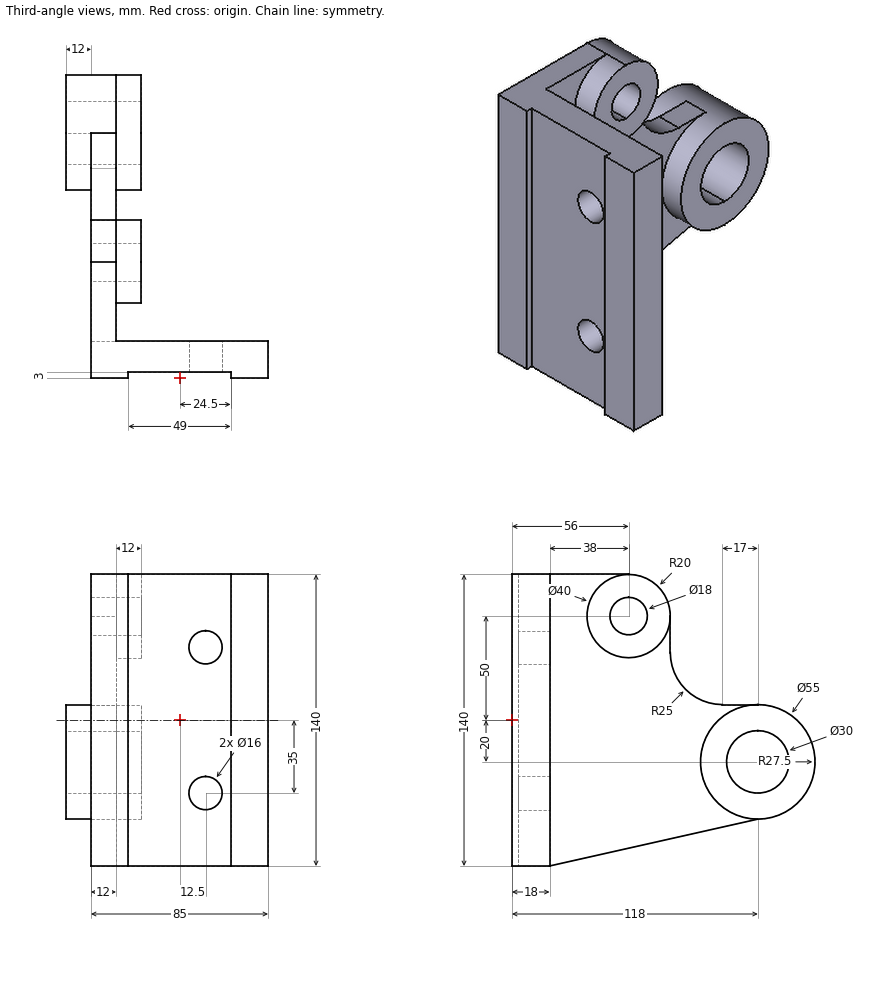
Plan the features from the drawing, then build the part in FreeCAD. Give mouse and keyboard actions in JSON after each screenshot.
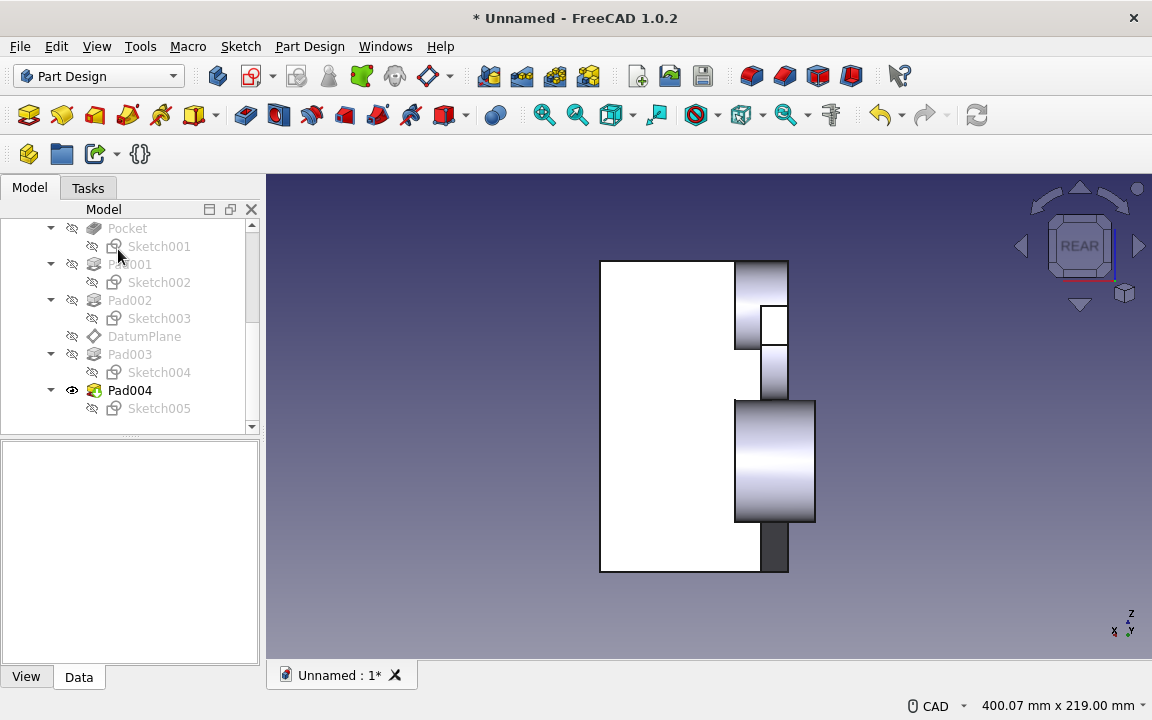
{"action": "left_click", "coordinate": [681, 371]}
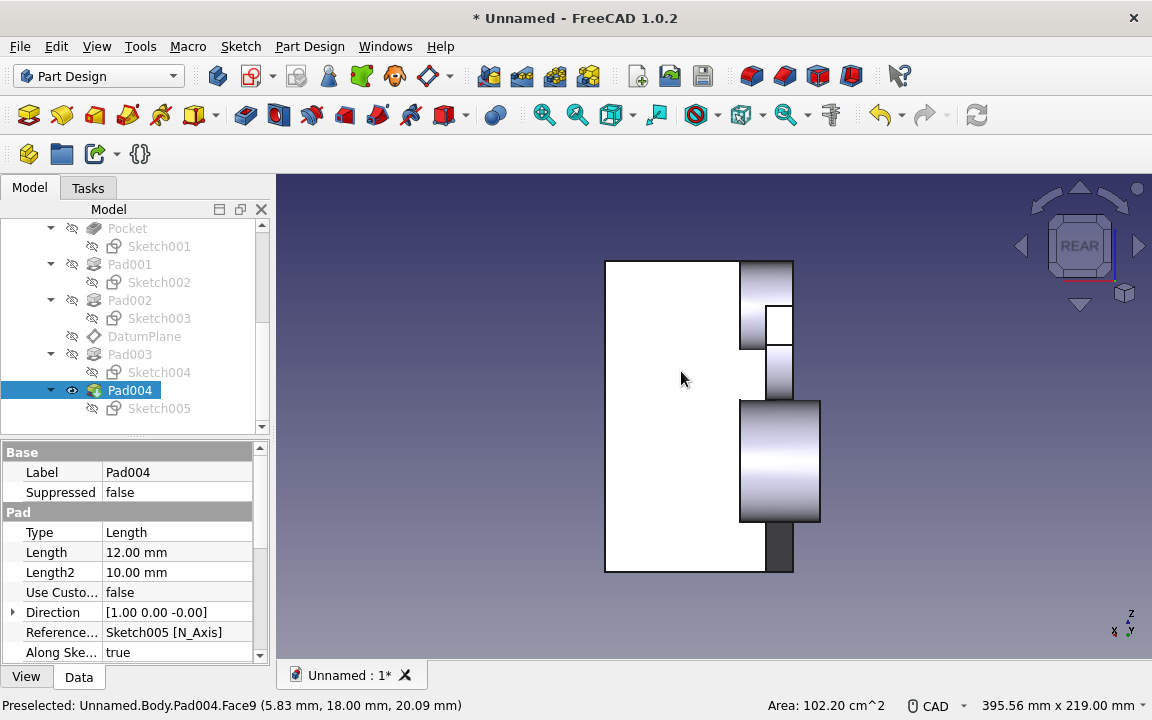
{"action": "left_click", "coordinate": [250, 76]}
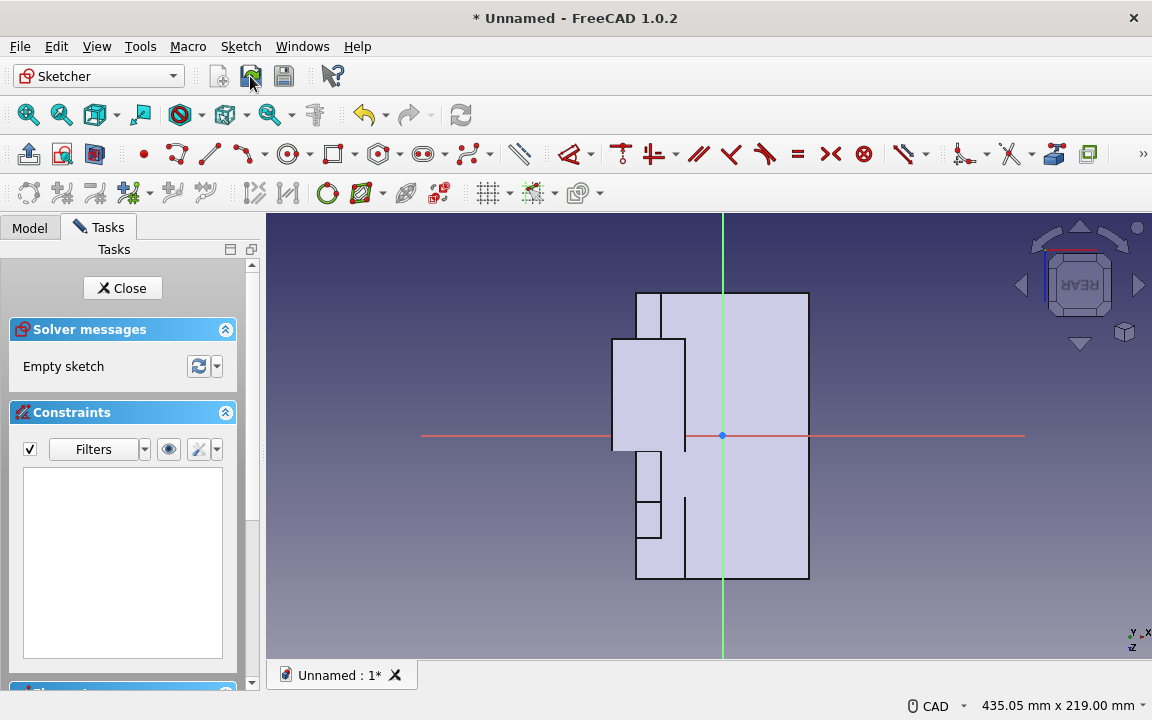
{"action": "left_click", "coordinate": [95, 154]}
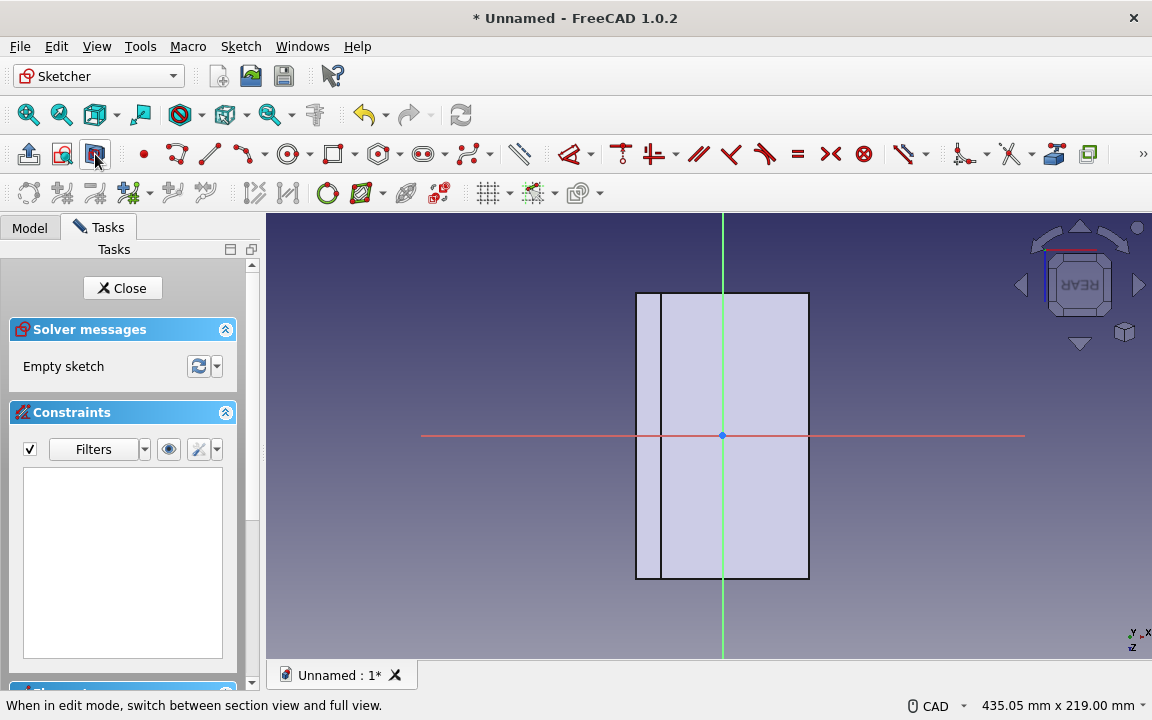
{"action": "scroll", "coordinate": [954, 436], "scroll_direction": "up", "scroll_amount": 2}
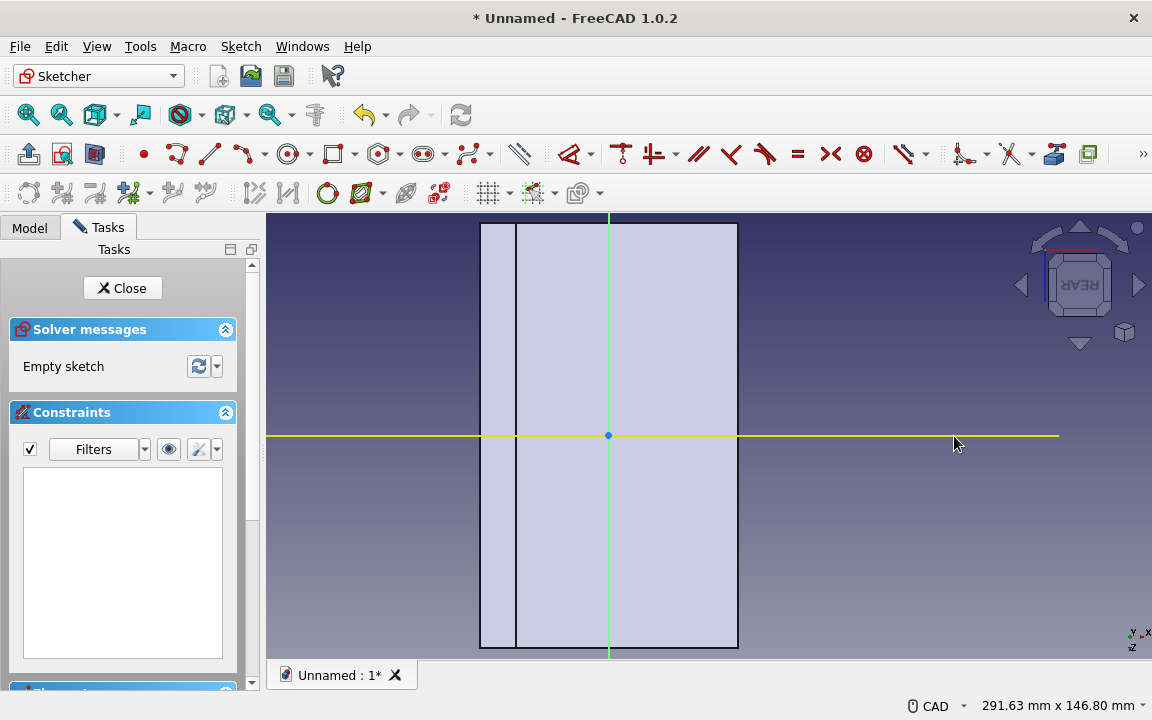
{"action": "key", "text": "g c"}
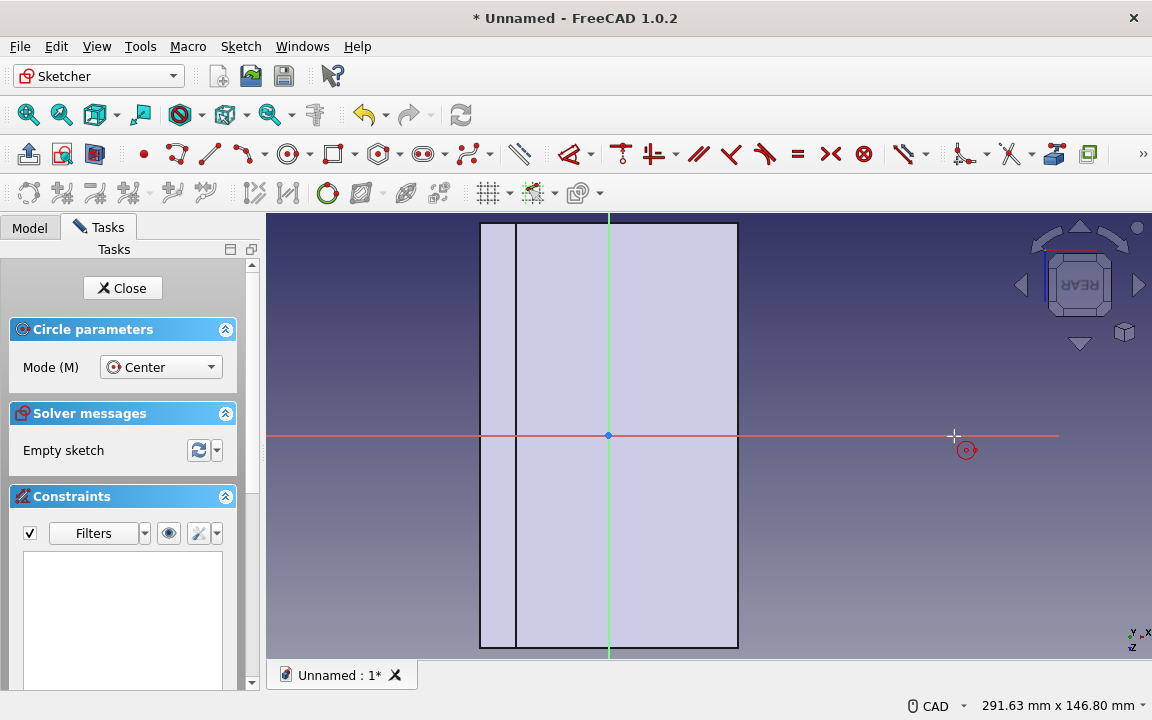
{"action": "left_click", "coordinate": [647, 329]}
{"action": "mouse_move", "coordinate": [664, 312]}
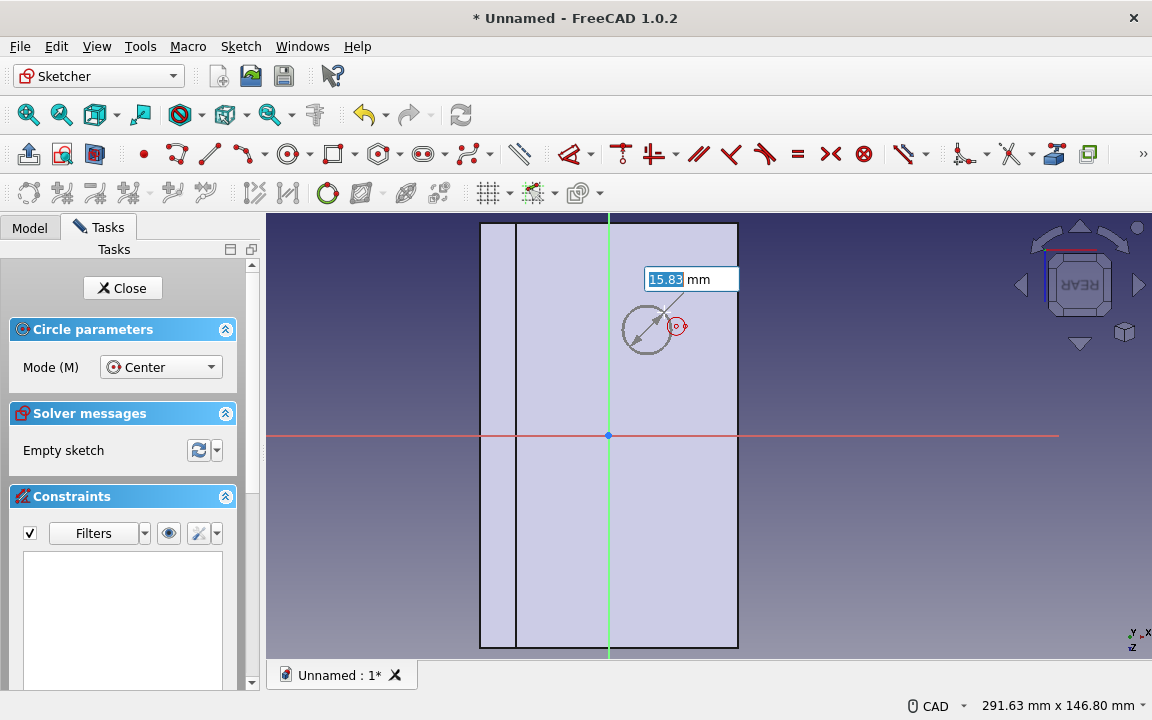
{"action": "type", "text": "16"}
{"action": "key", "text": "Return"}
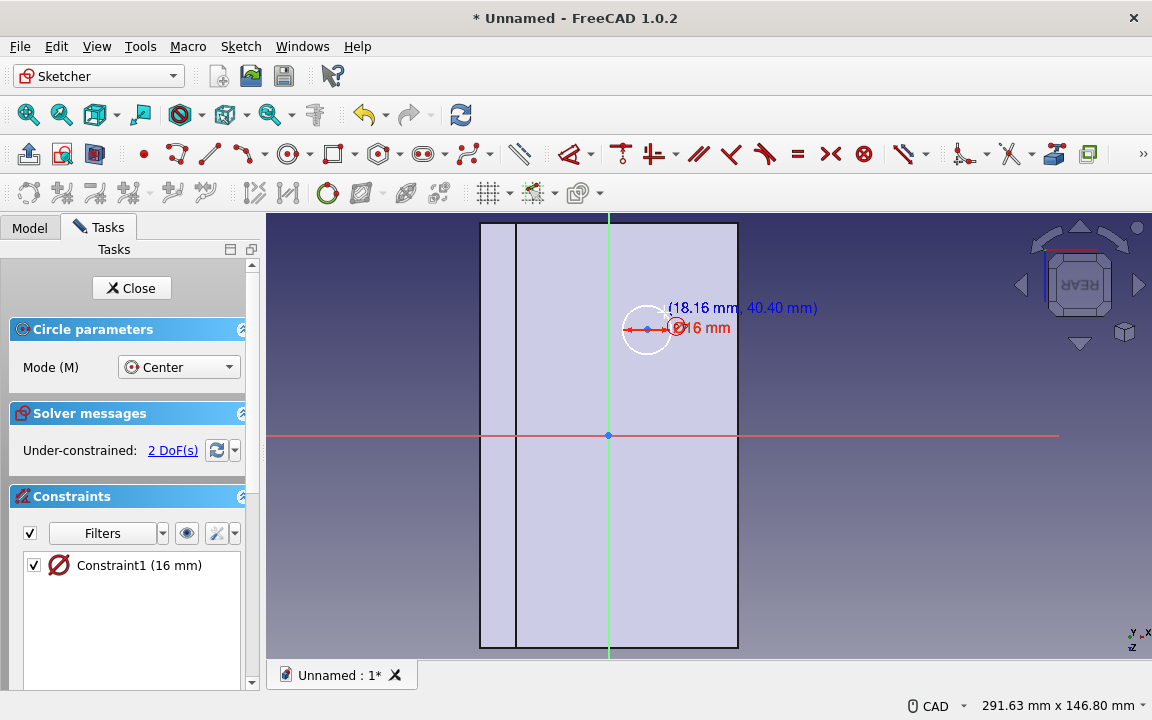
{"action": "left_click", "coordinate": [647, 542]}
{"action": "mouse_move", "coordinate": [664, 525]}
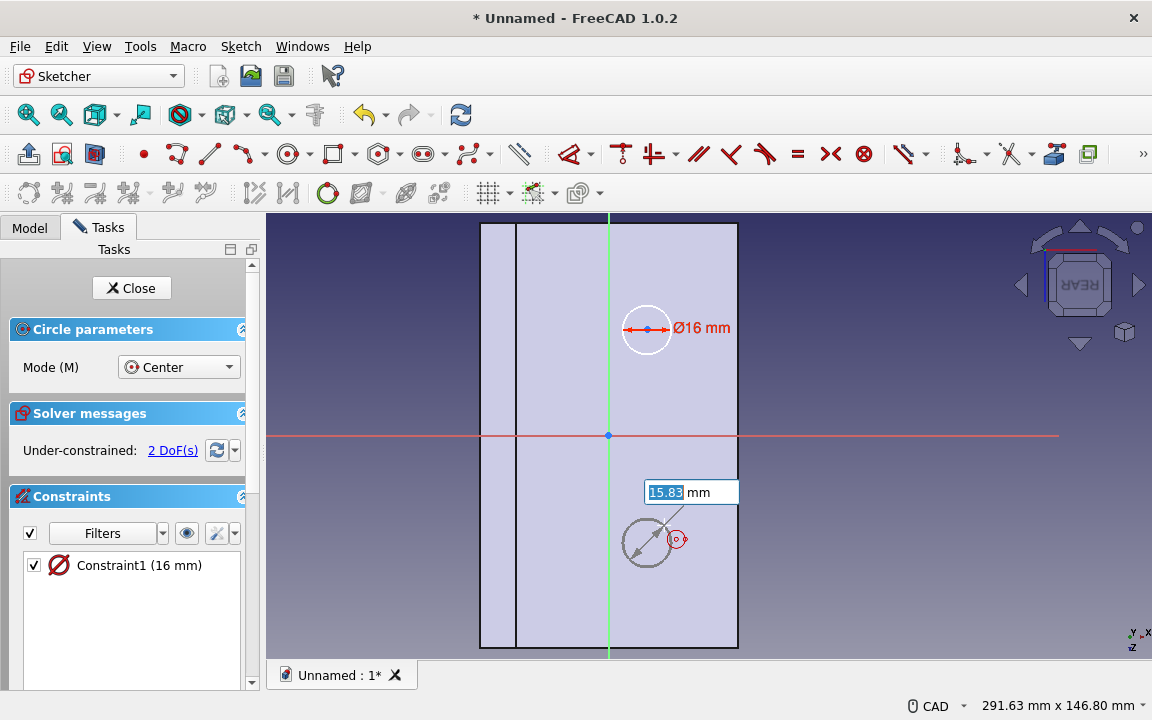
{"action": "type", "text": "16"}
{"action": "key", "text": "Return"}
{"action": "key", "text": "Escape"}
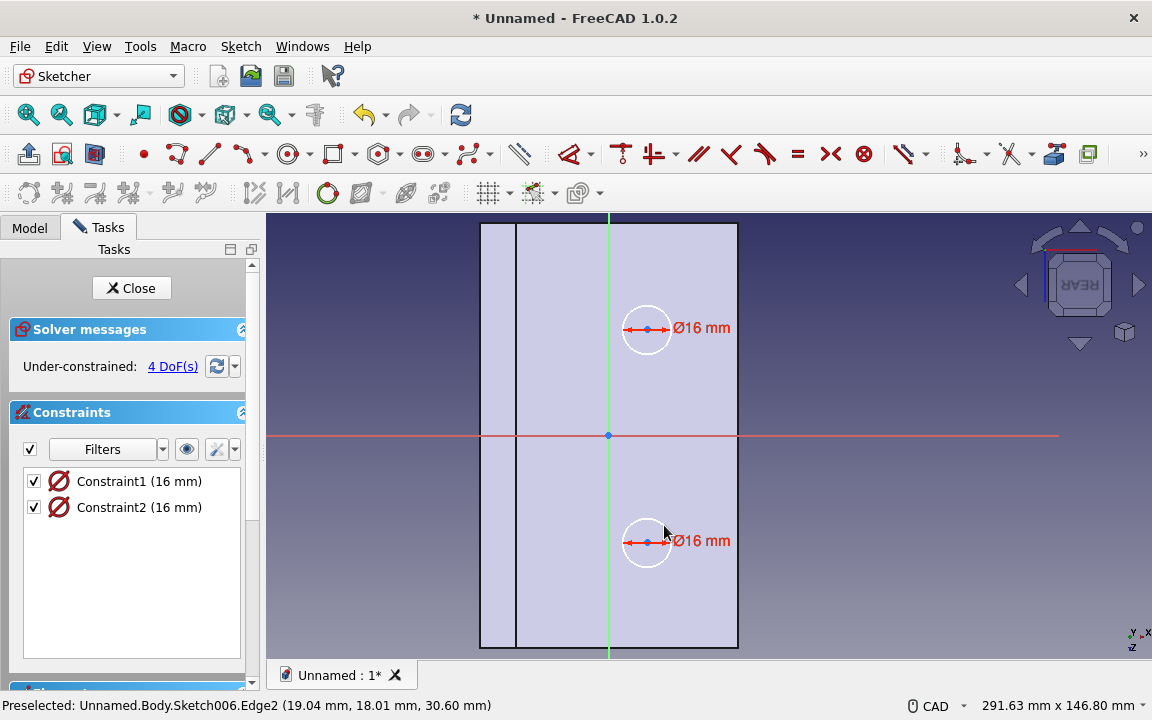
{"action": "left_click", "coordinate": [647, 330]}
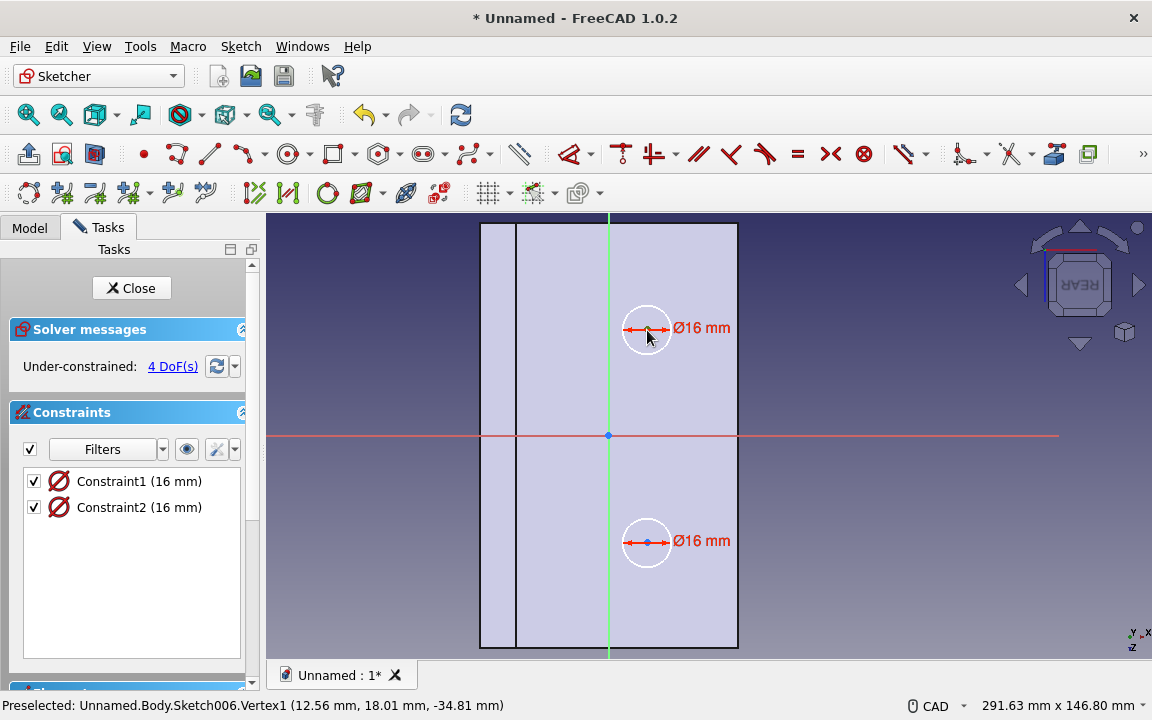
{"action": "left_click", "coordinate": [647, 543]}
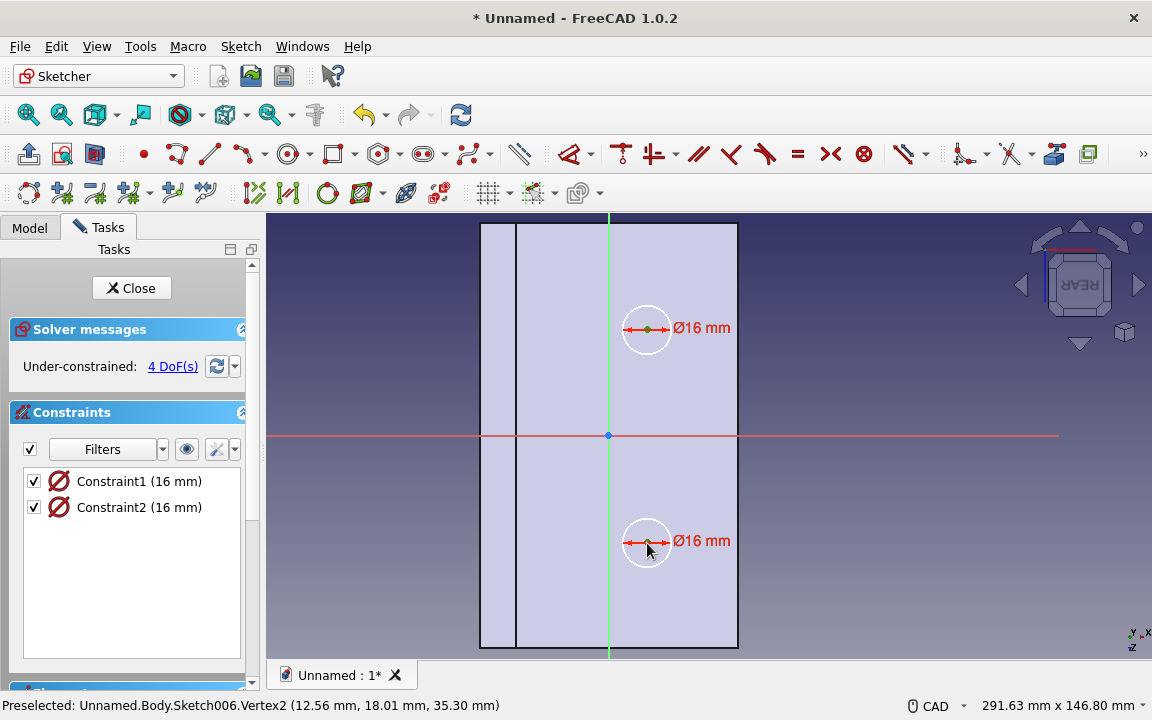
{"action": "left_click", "coordinate": [344, 436]}